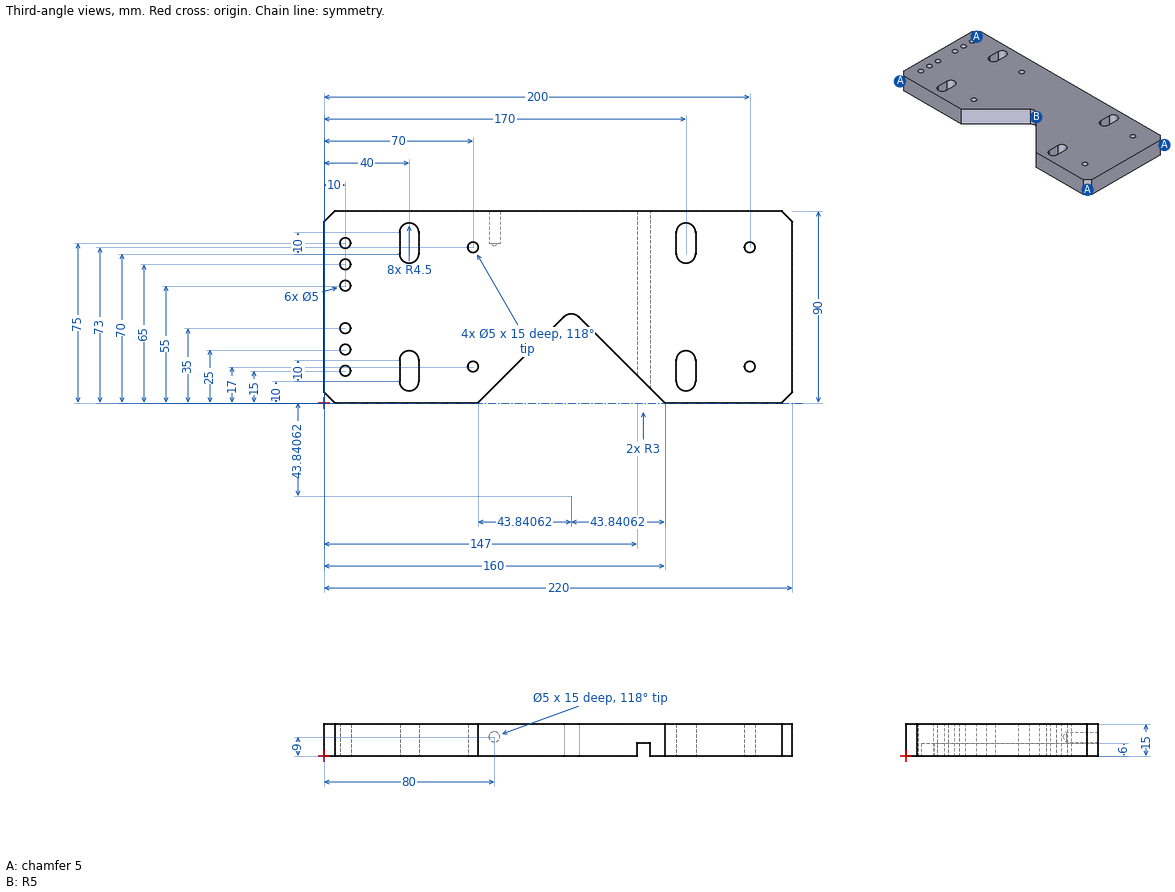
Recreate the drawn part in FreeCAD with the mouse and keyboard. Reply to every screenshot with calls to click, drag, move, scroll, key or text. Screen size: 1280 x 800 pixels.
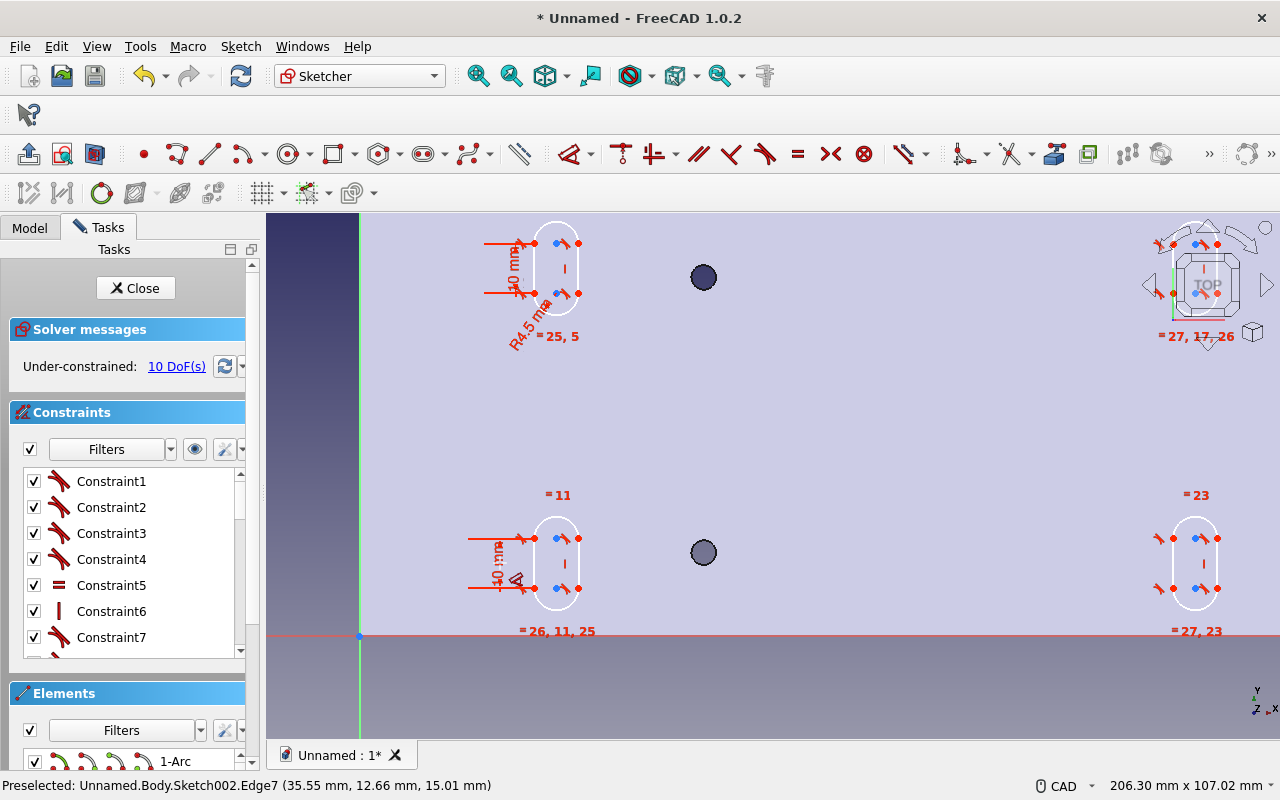
scroll(534, 572, down, 2)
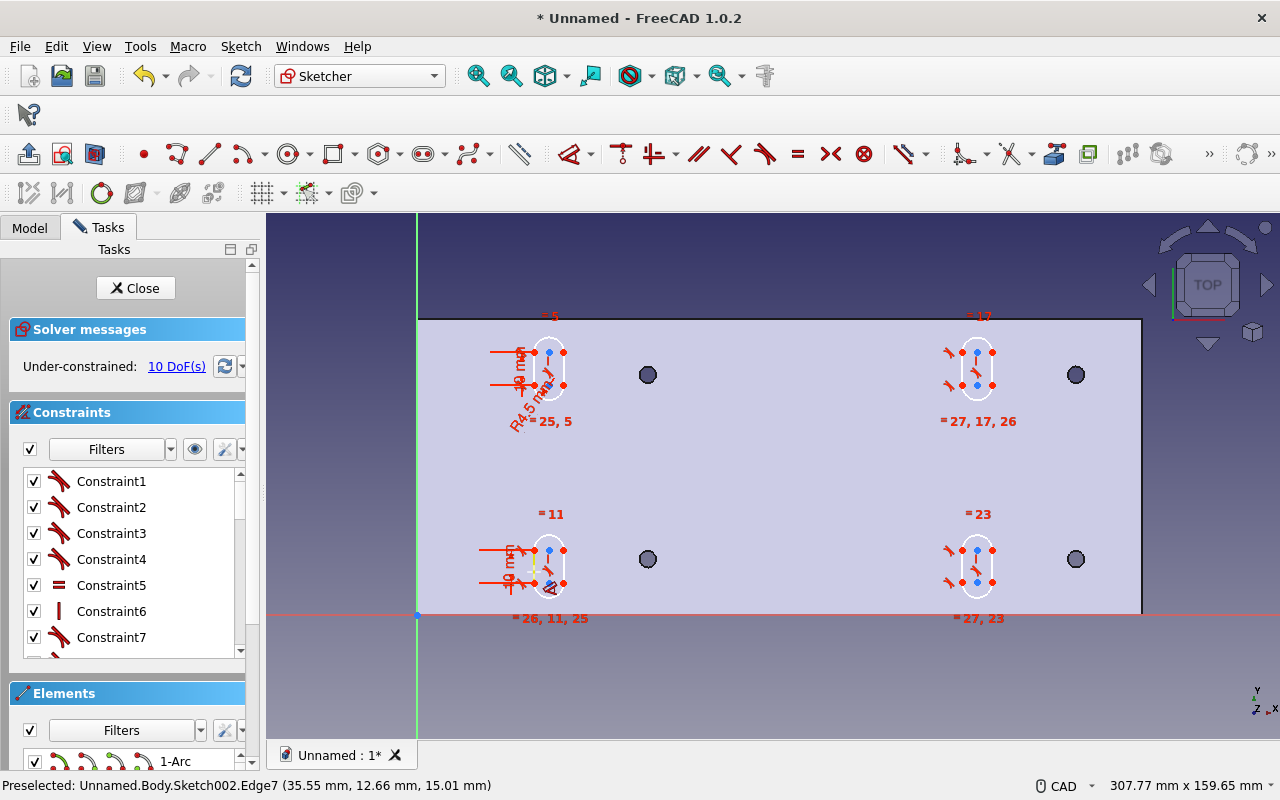
scroll(962, 375, up, 2)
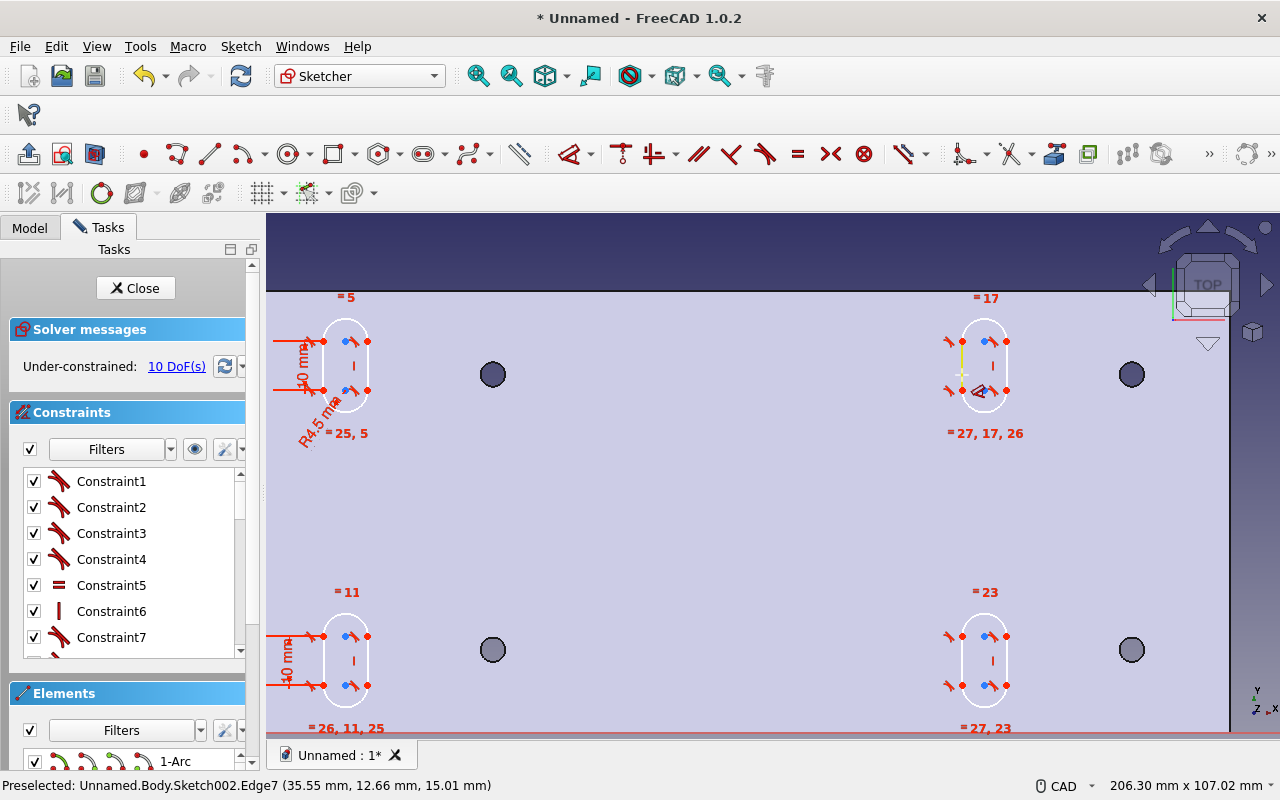
click(962, 376)
click(928, 366)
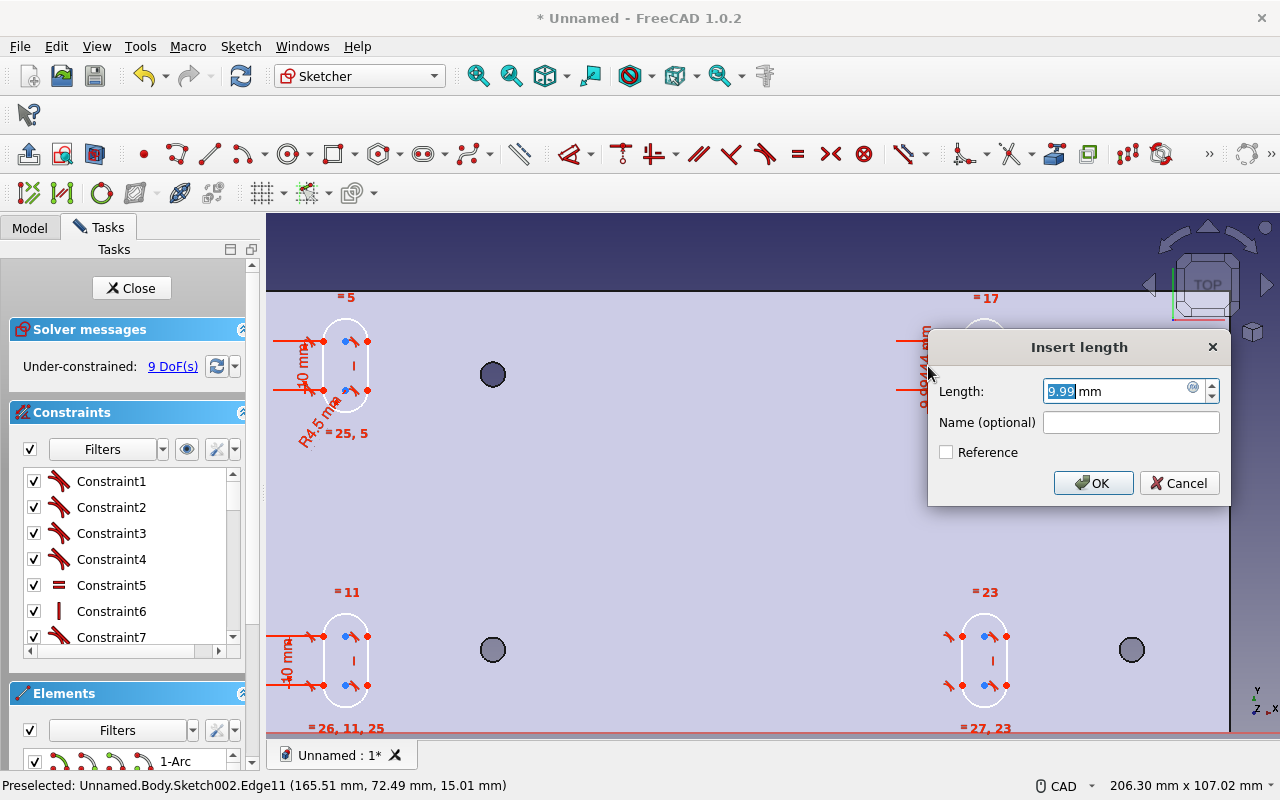
text(10)
key(Return)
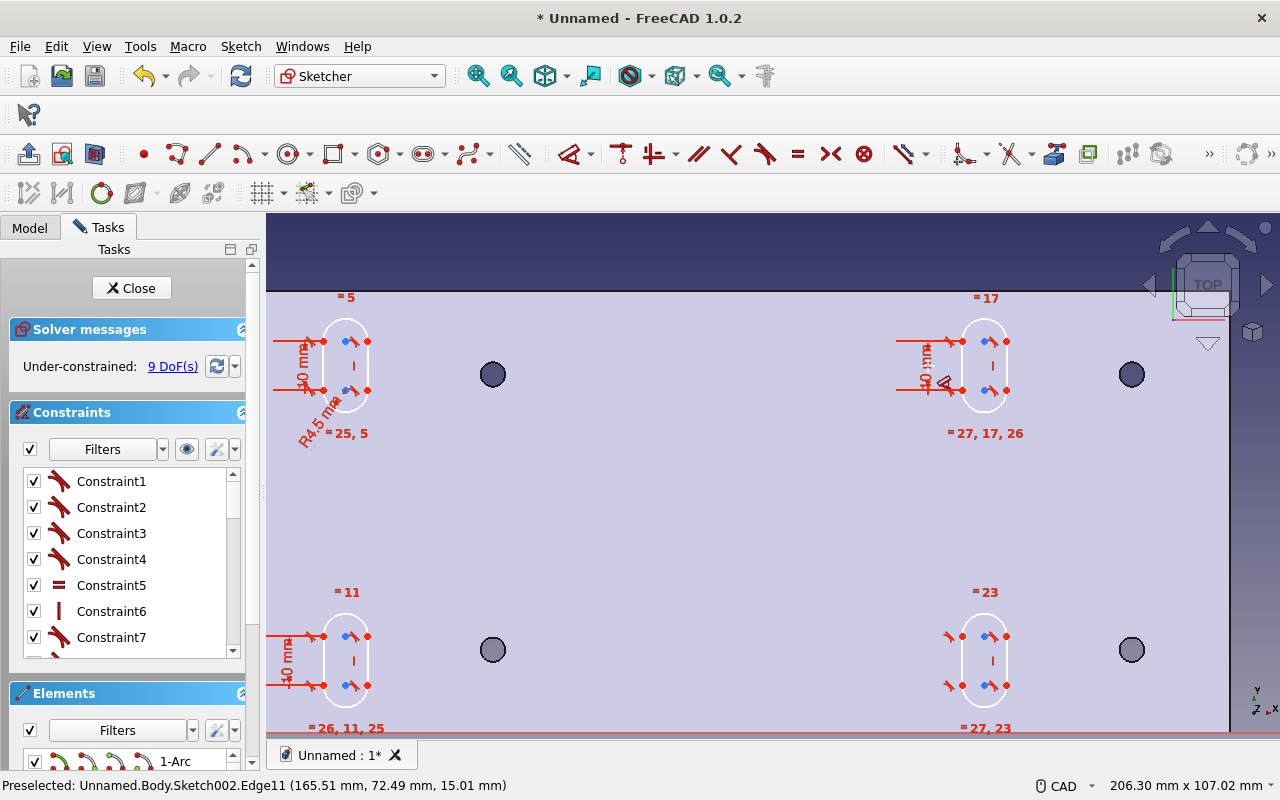
click(962, 670)
click(928, 661)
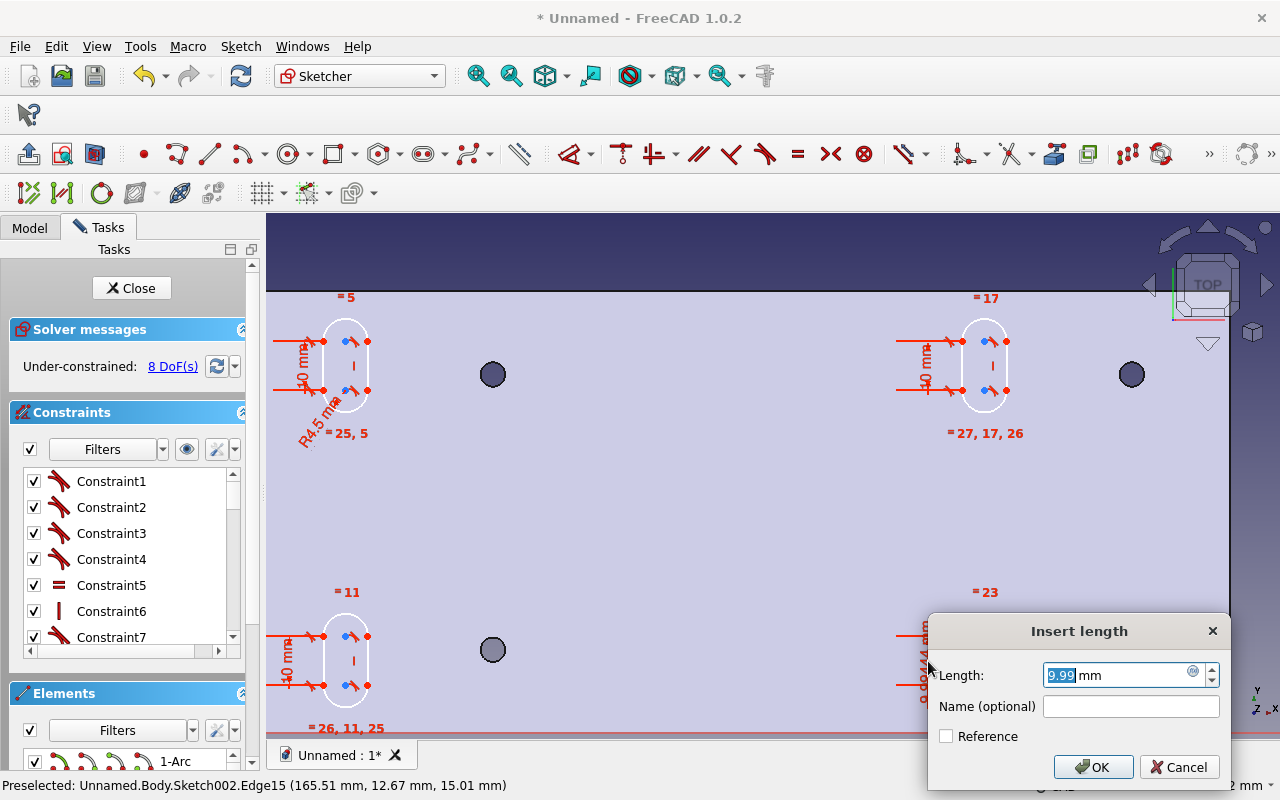
text(10)
key(Return)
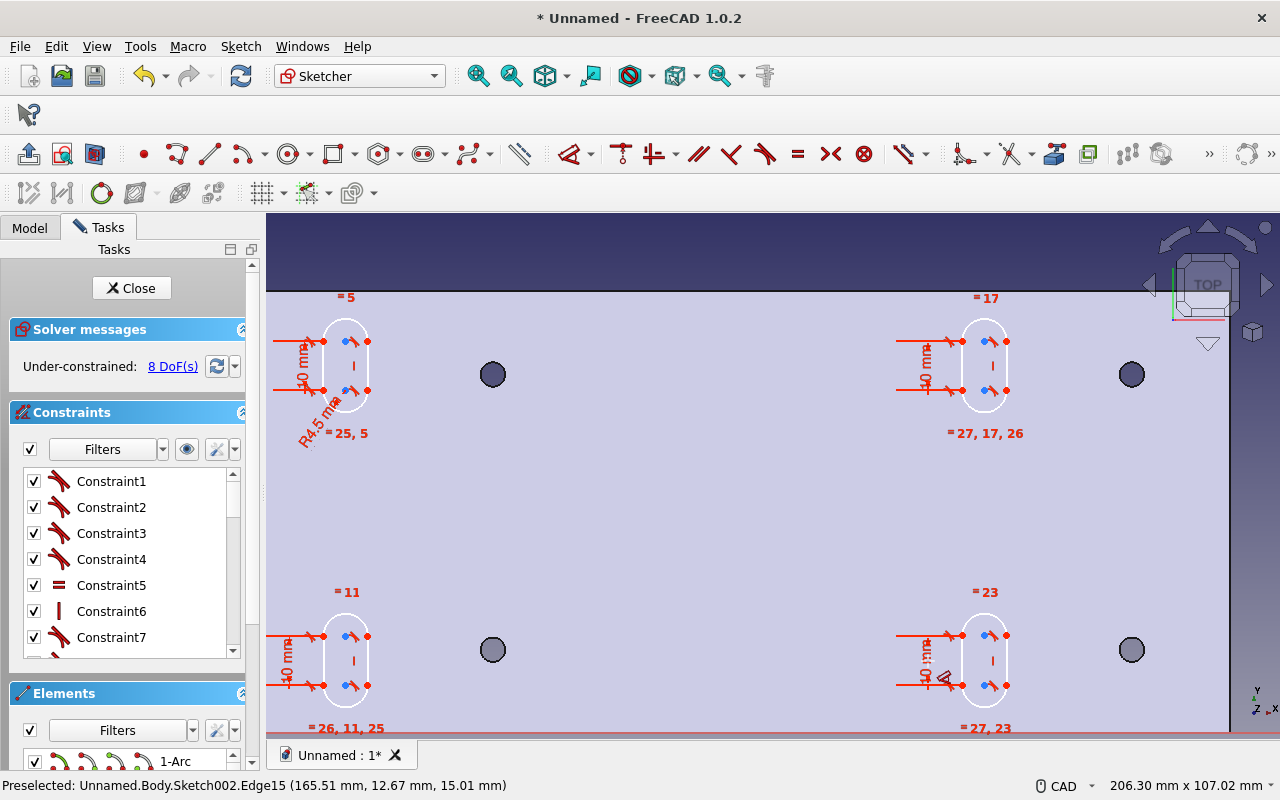
click(323, 390)
click(357, 551)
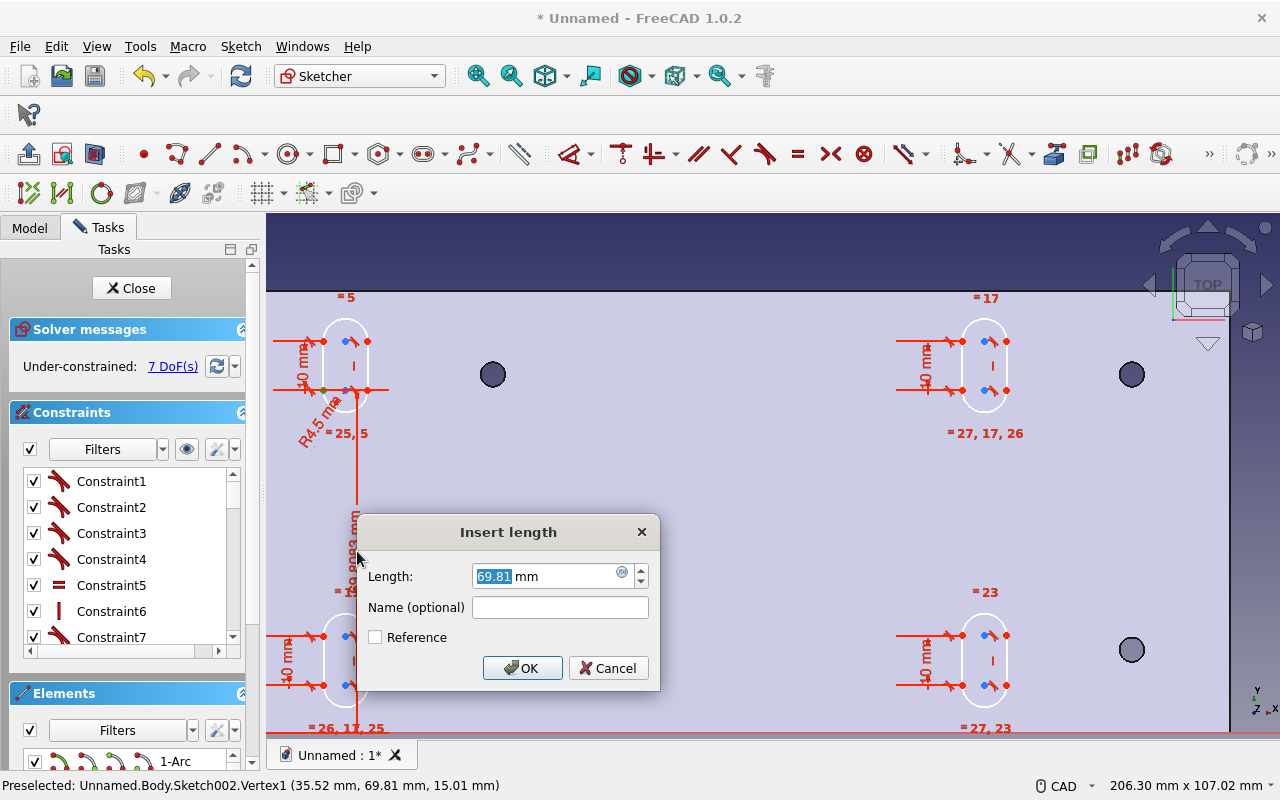
text(70)
key(Return)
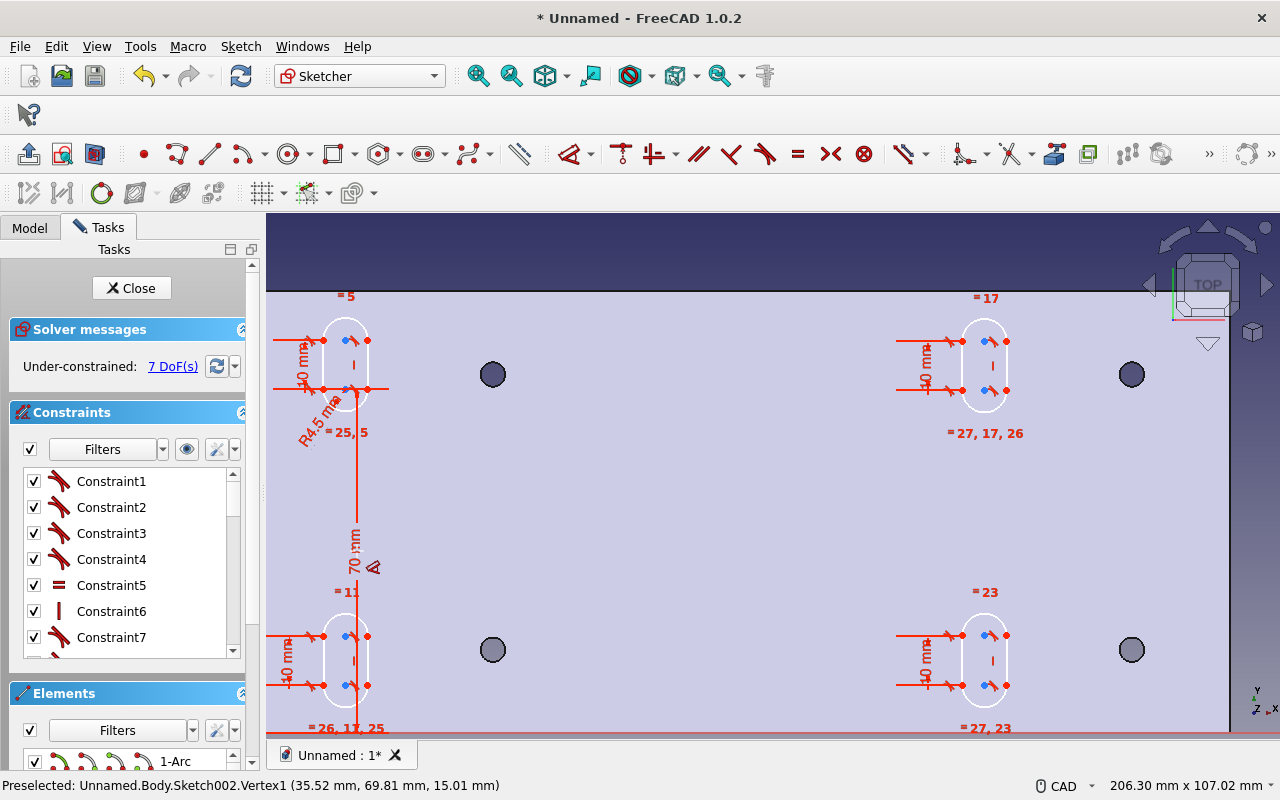
click(324, 685)
click(382, 698)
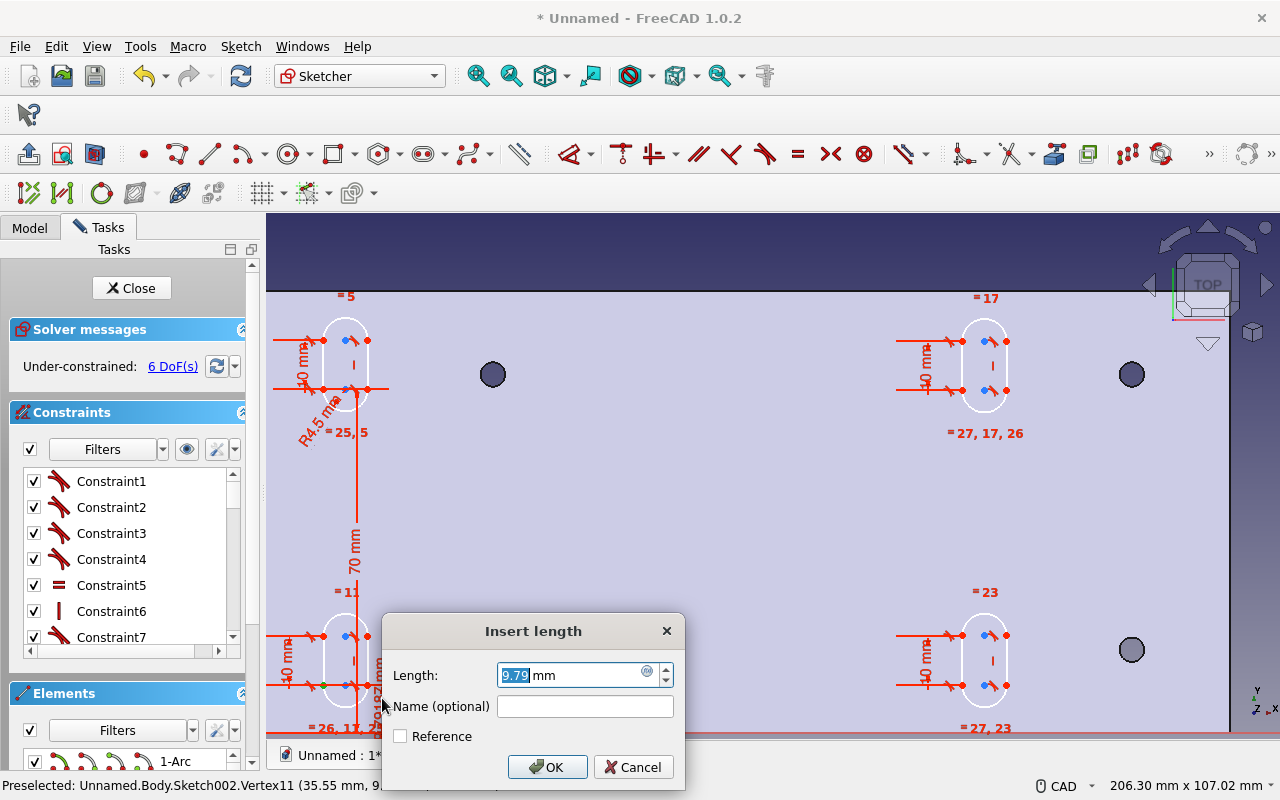
text(10)
key(Return)